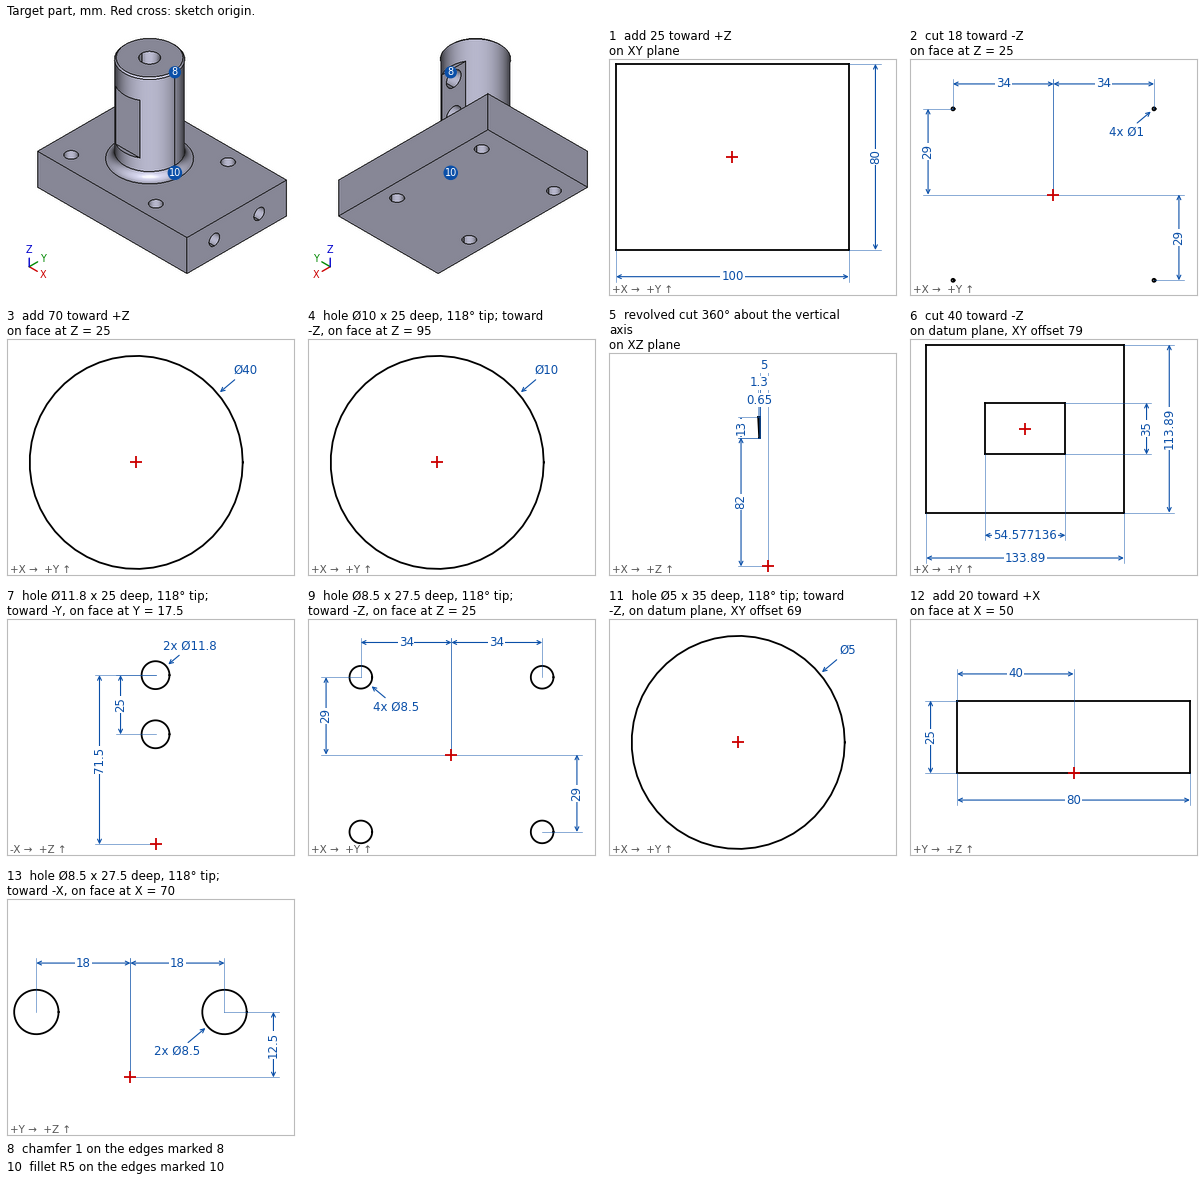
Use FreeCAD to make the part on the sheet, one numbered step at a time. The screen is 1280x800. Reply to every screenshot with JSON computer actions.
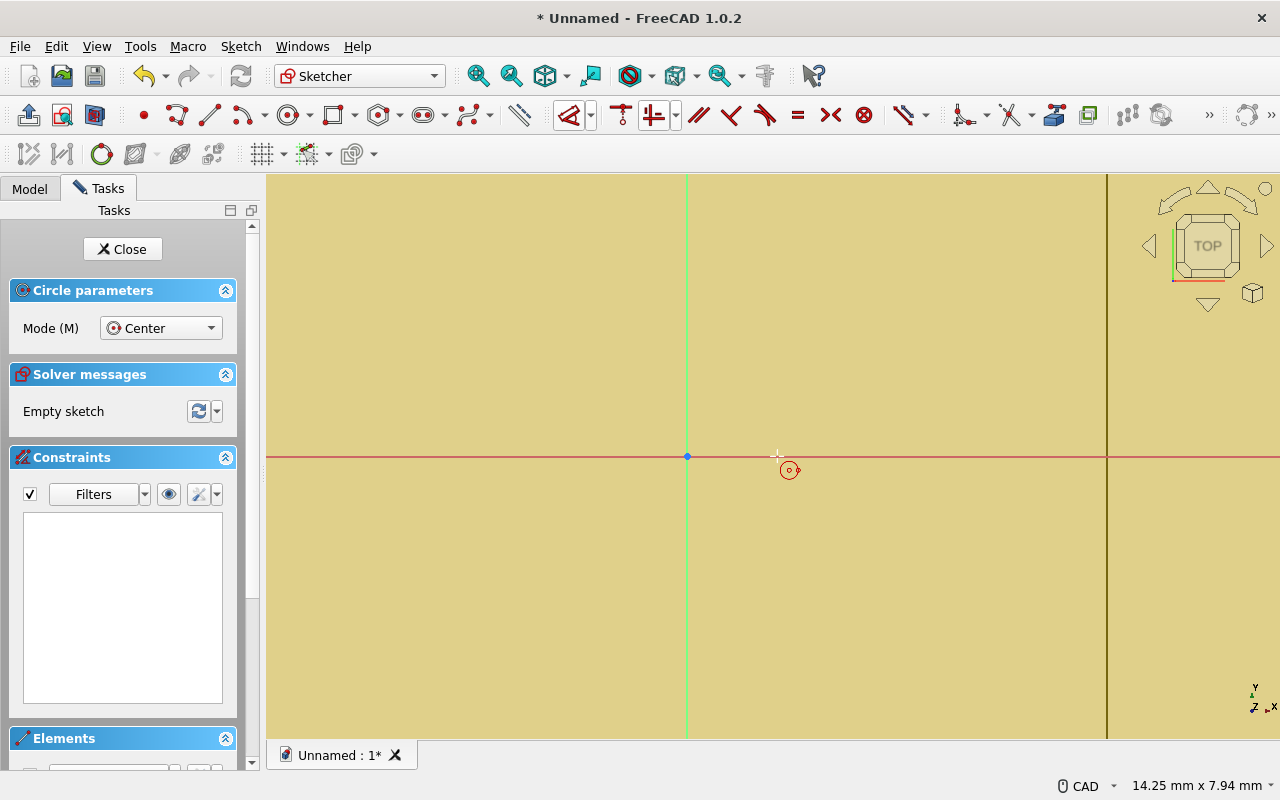
{"action": "left_click", "coordinate": [687, 456]}
{"action": "mouse_move", "coordinate": [813, 331]}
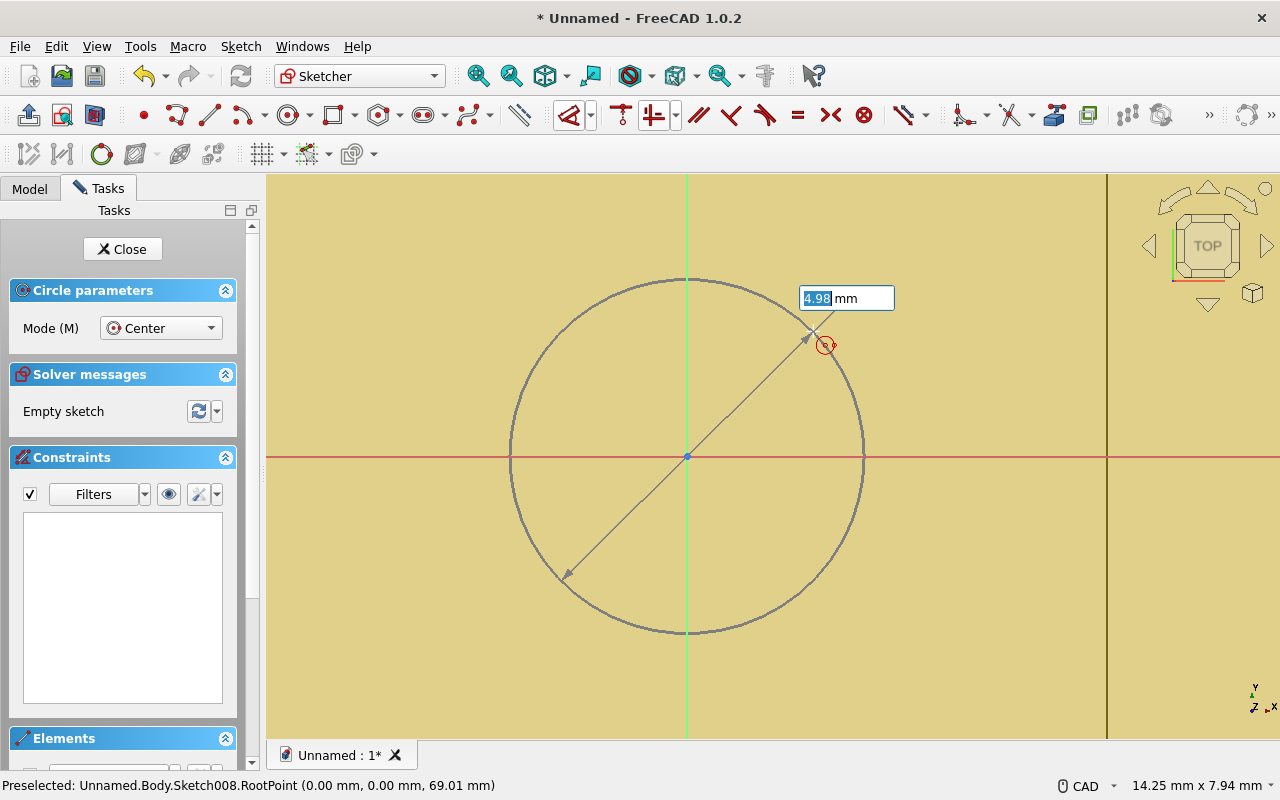
{"action": "type", "text": "5"}
{"action": "key", "text": "Return"}
{"action": "key", "text": "Escape"}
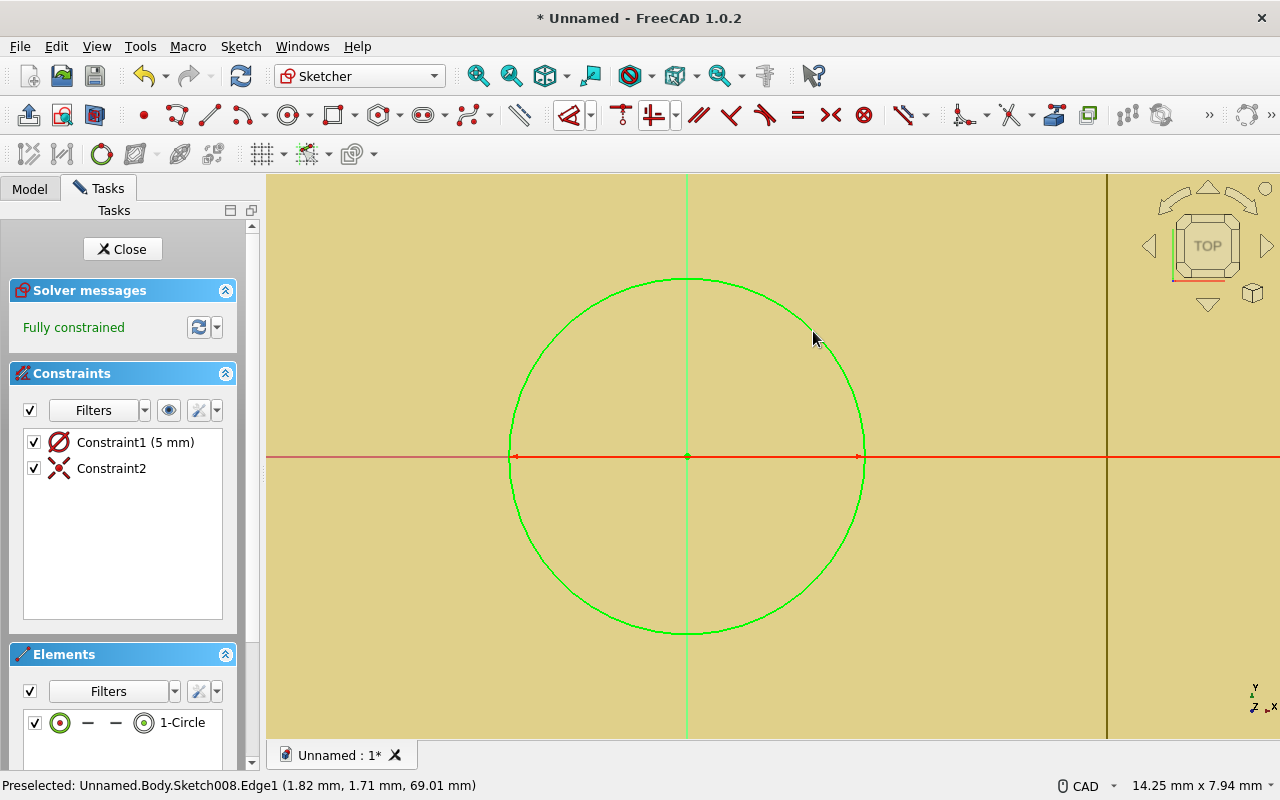
{"action": "left_click", "coordinate": [123, 249]}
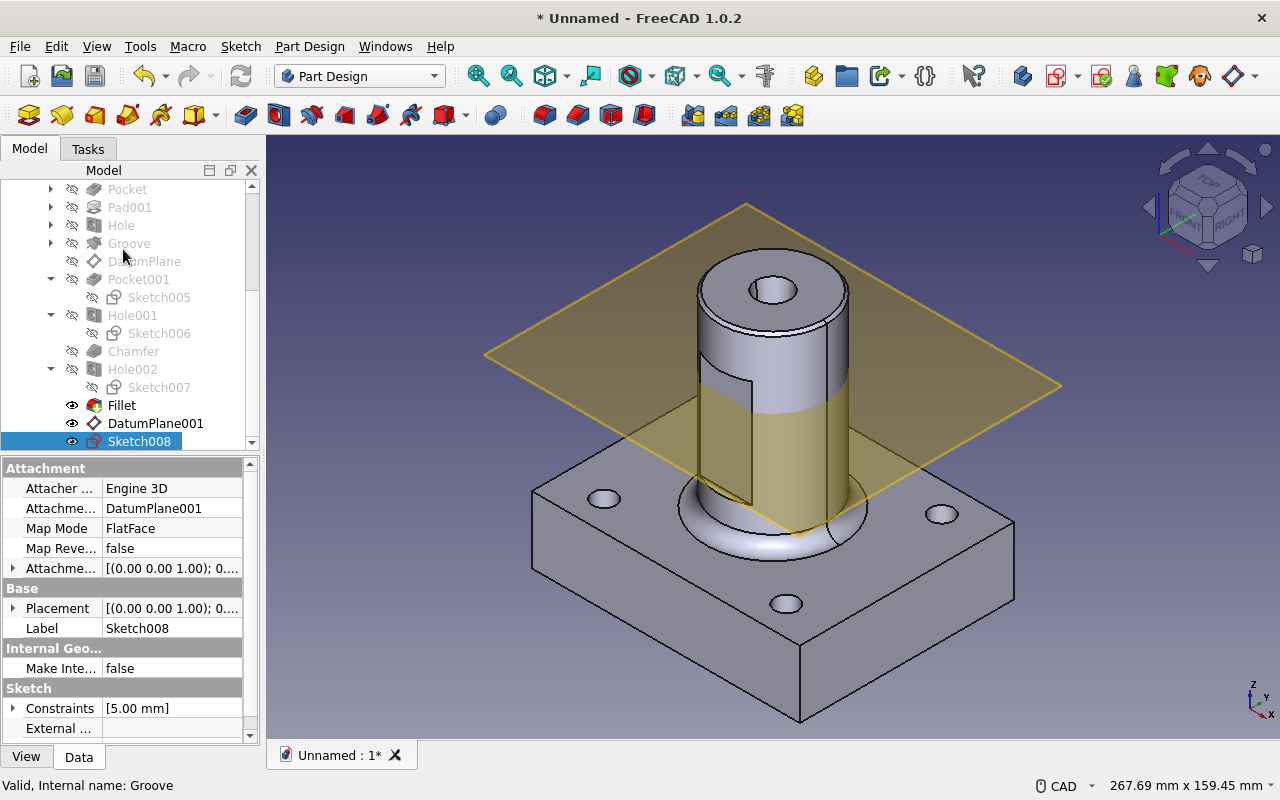
{"action": "left_click", "coordinate": [279, 116]}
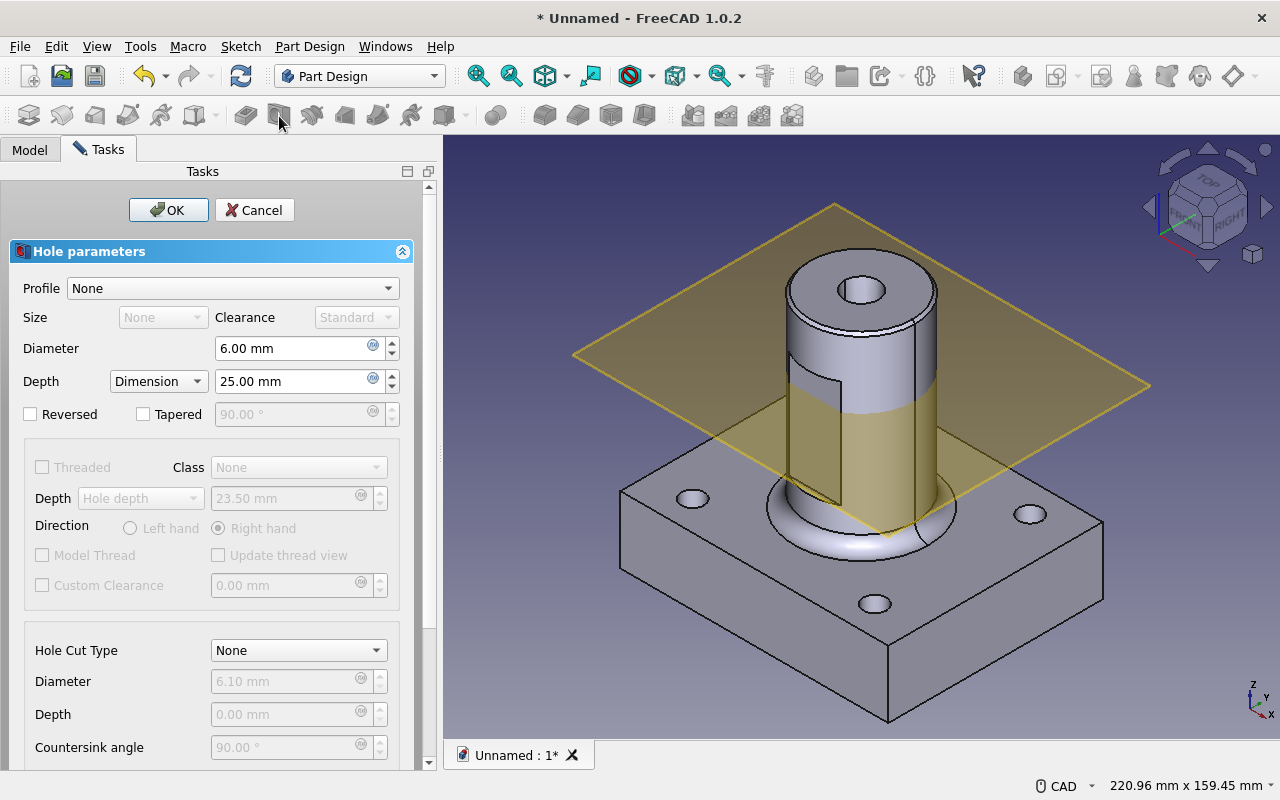
{"action": "triple_click", "coordinate": [300, 348]}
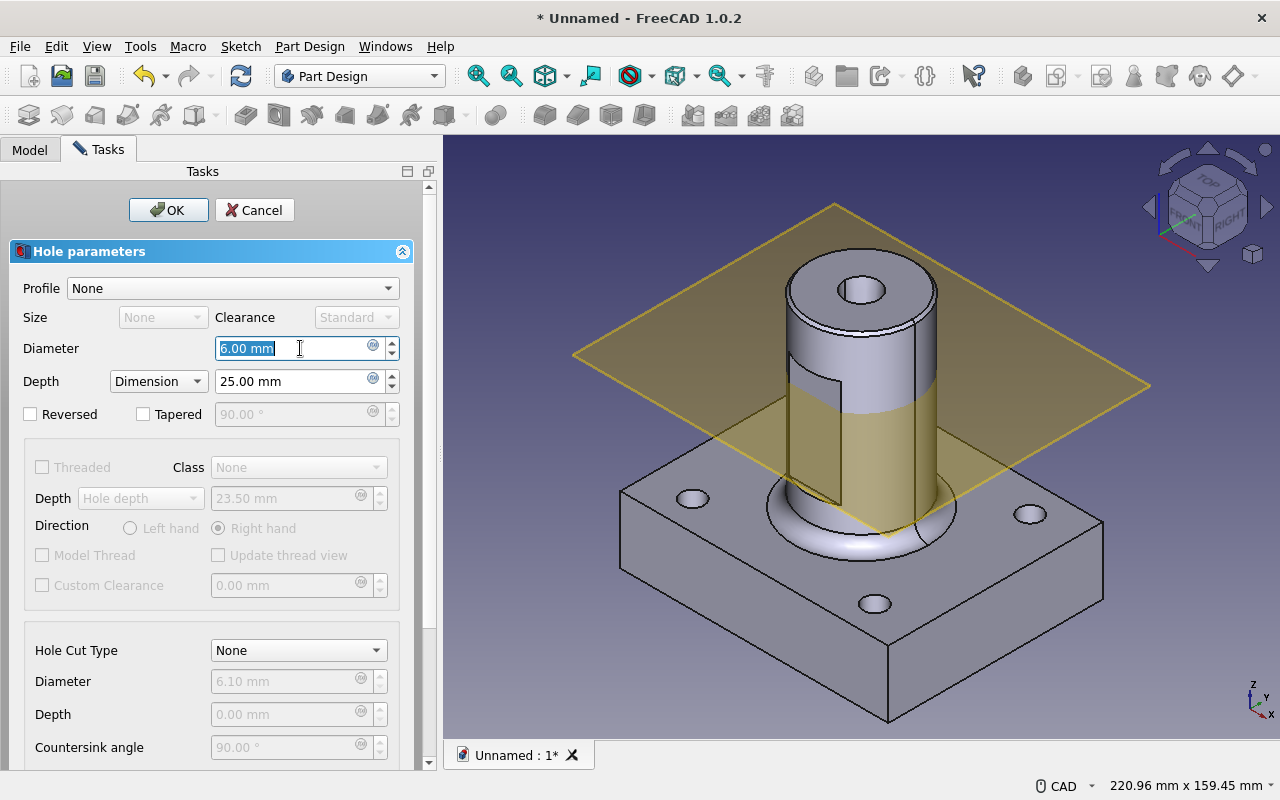
{"action": "type", "text": "5"}
{"action": "key", "text": "Tab"}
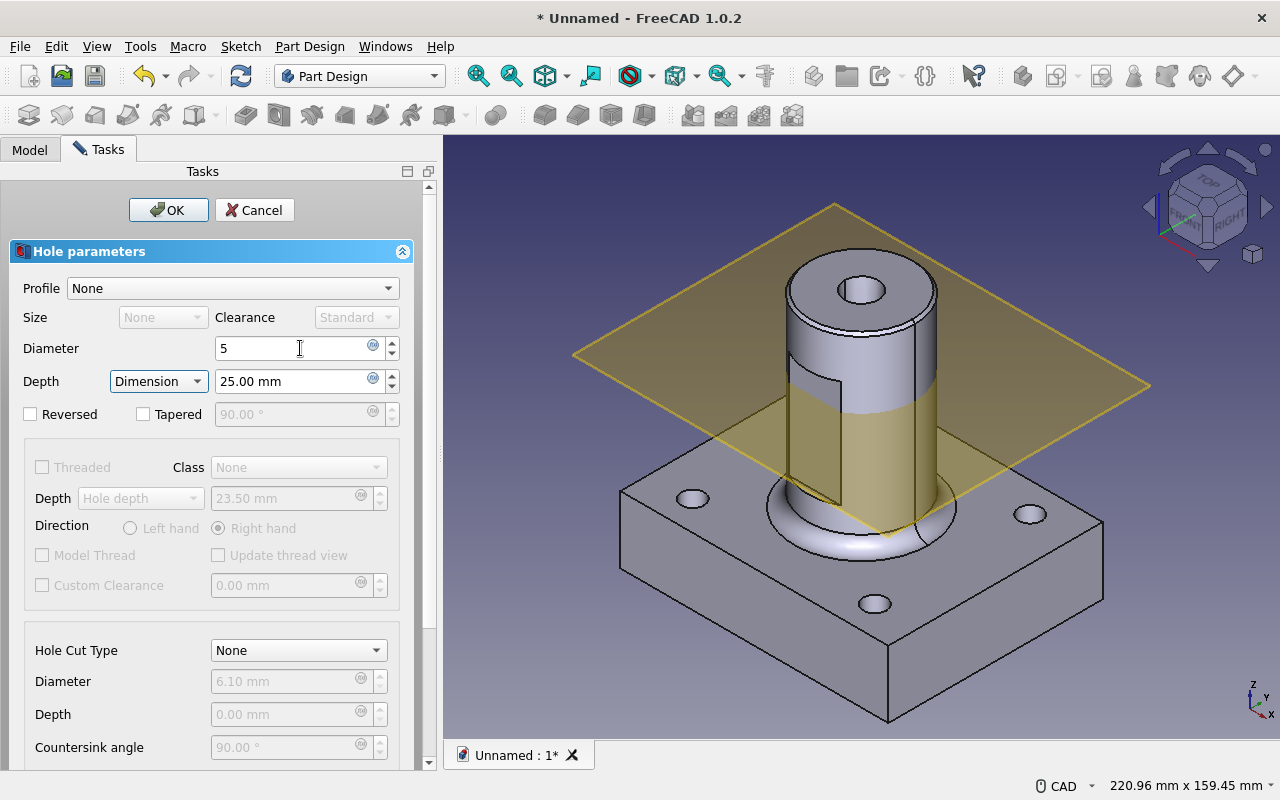
{"action": "triple_click", "coordinate": [300, 382]}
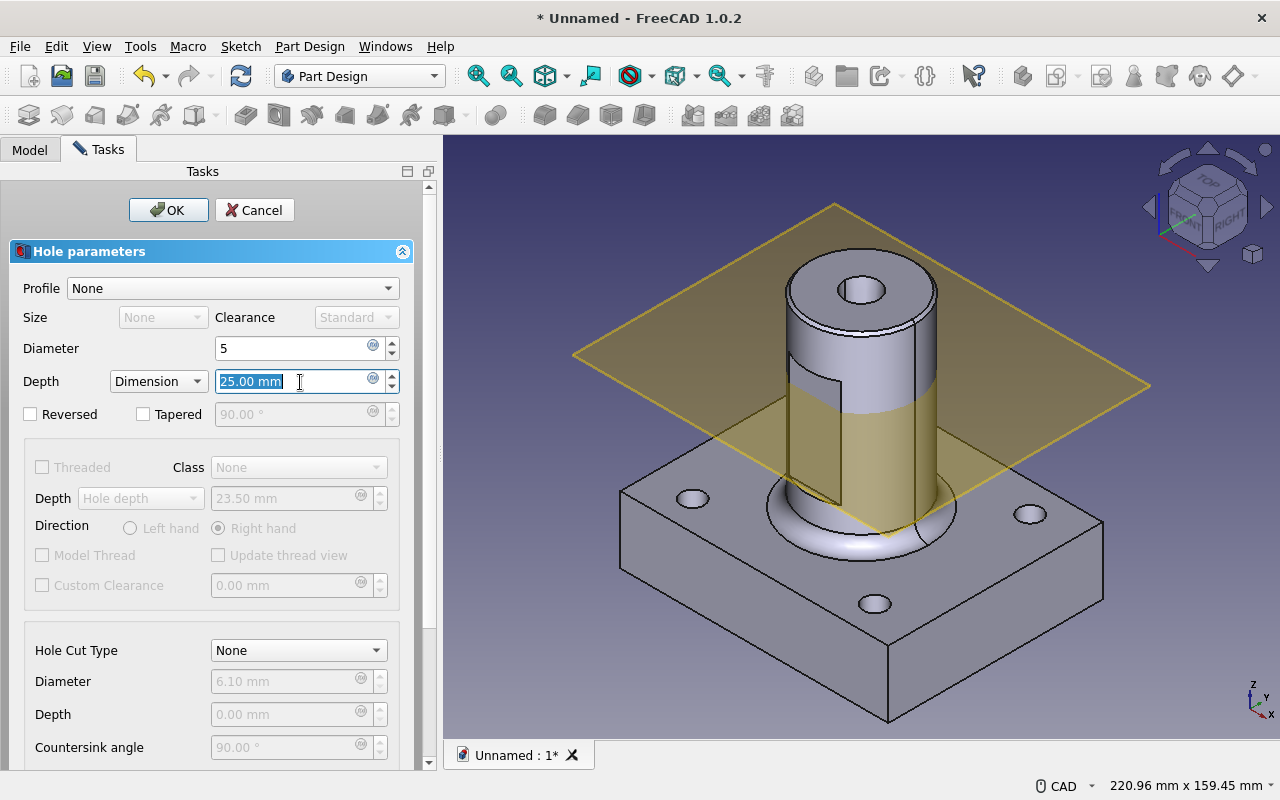
{"action": "type", "text": "35"}
{"action": "key", "text": "Tab"}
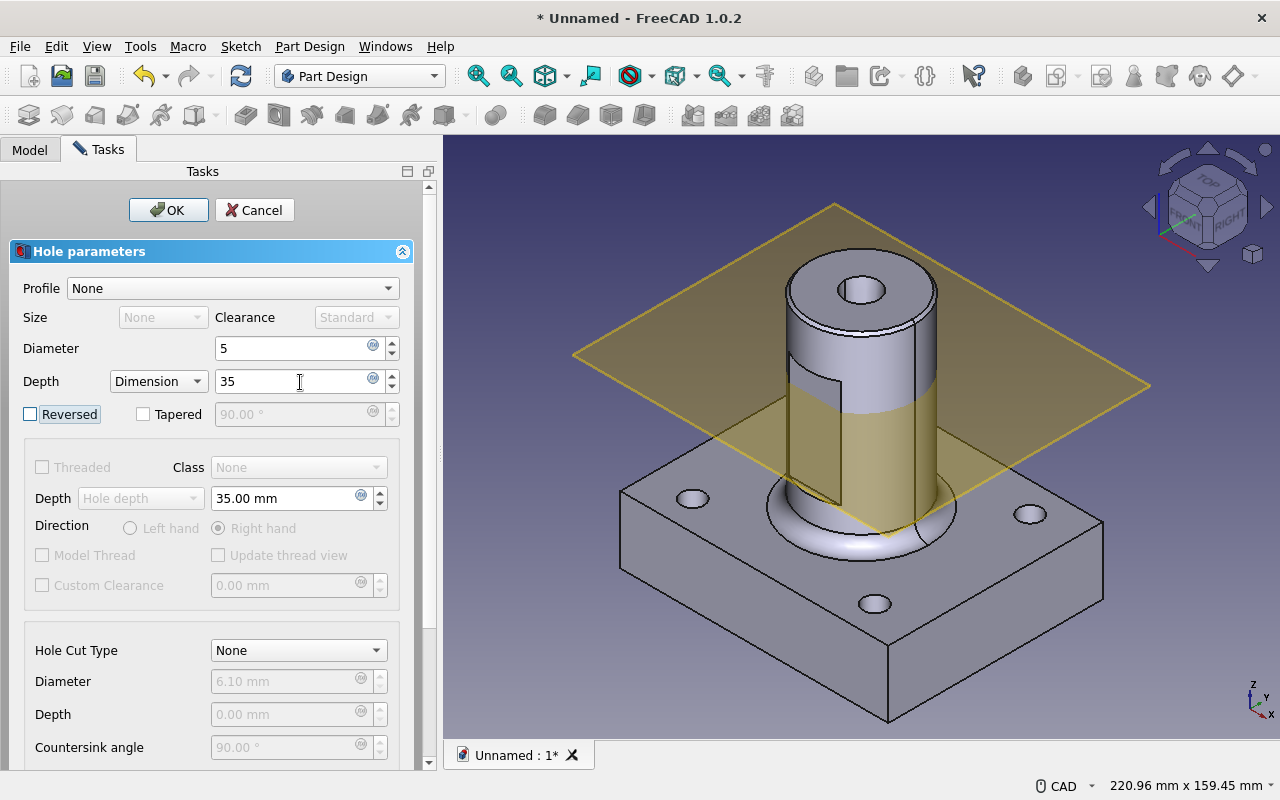
{"action": "left_click", "coordinate": [169, 210]}